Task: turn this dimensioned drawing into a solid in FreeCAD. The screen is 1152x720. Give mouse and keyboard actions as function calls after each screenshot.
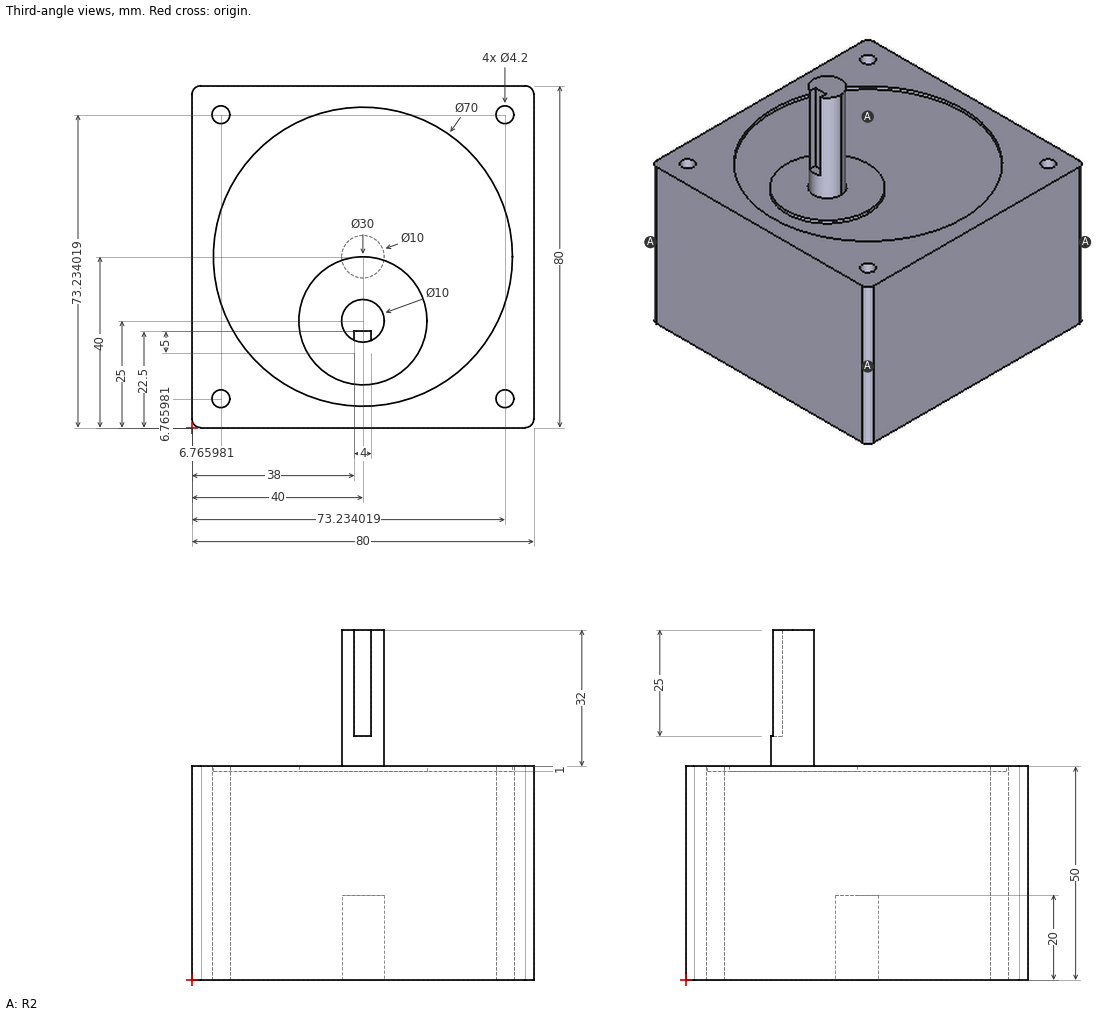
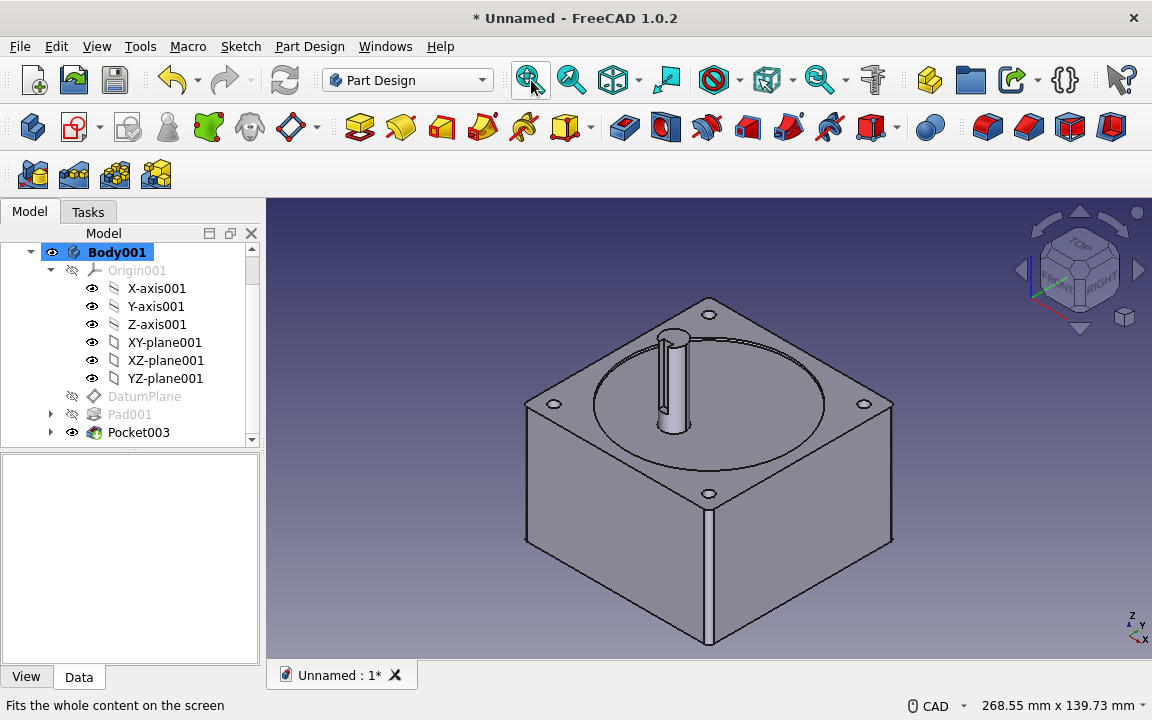
scroll(121, 338, down, 3)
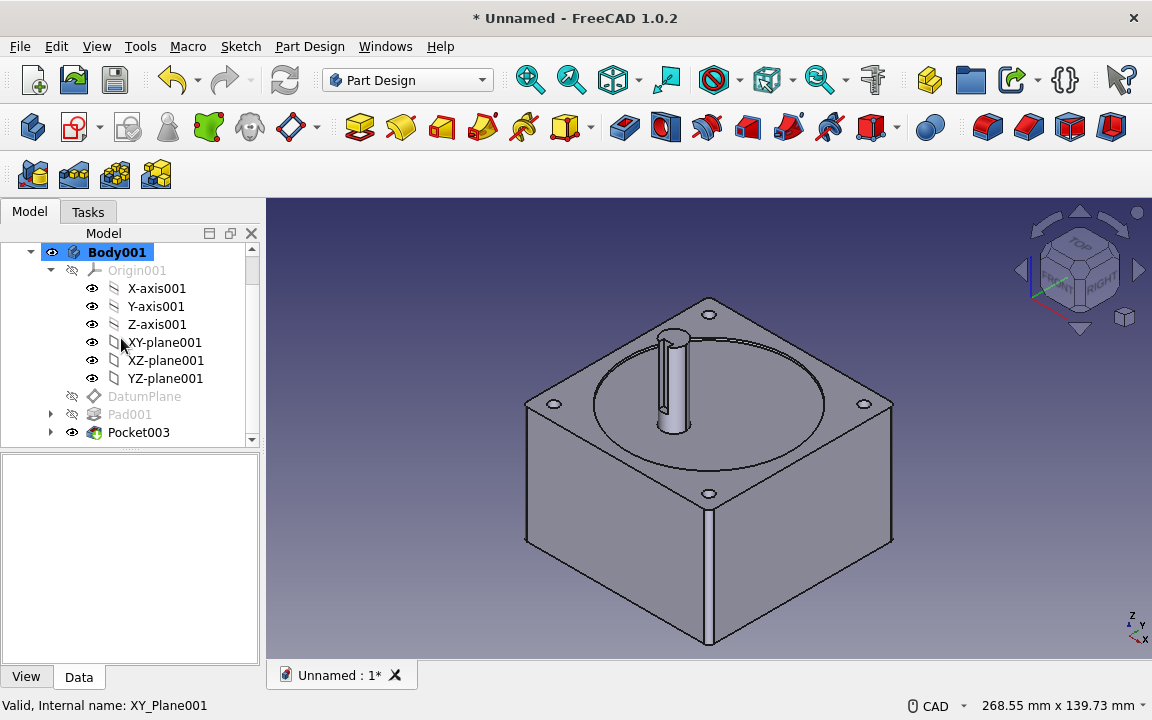
scroll(121, 338, up, 15)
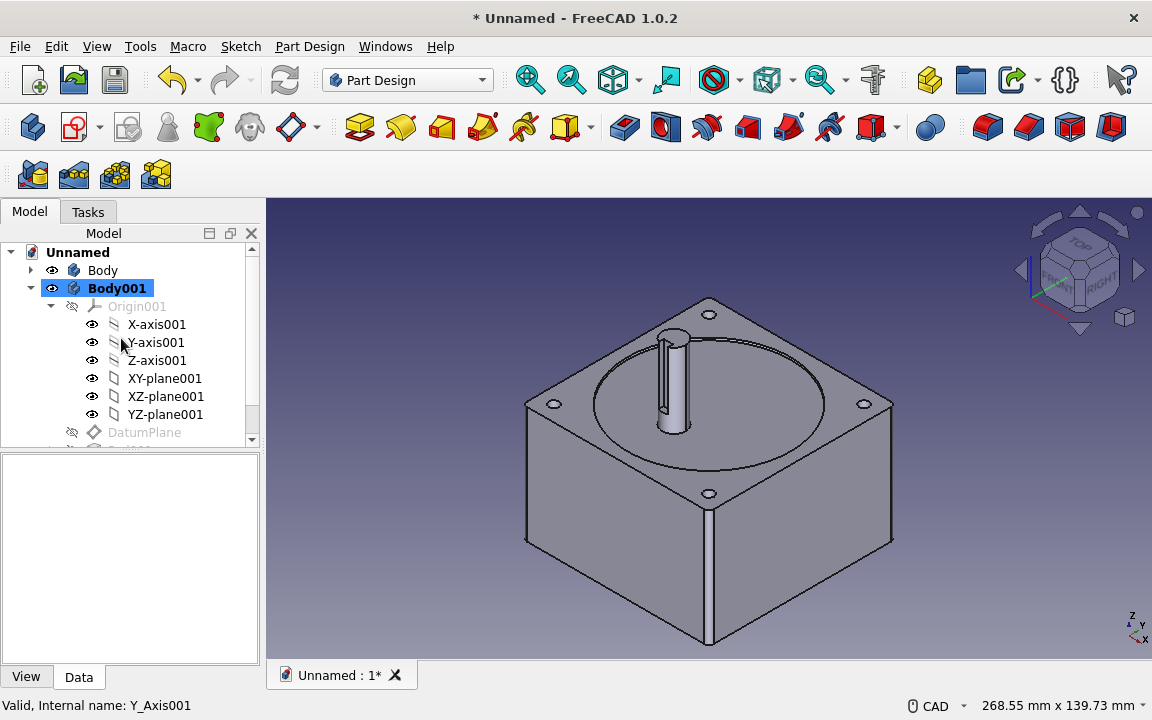
double_click(97, 270)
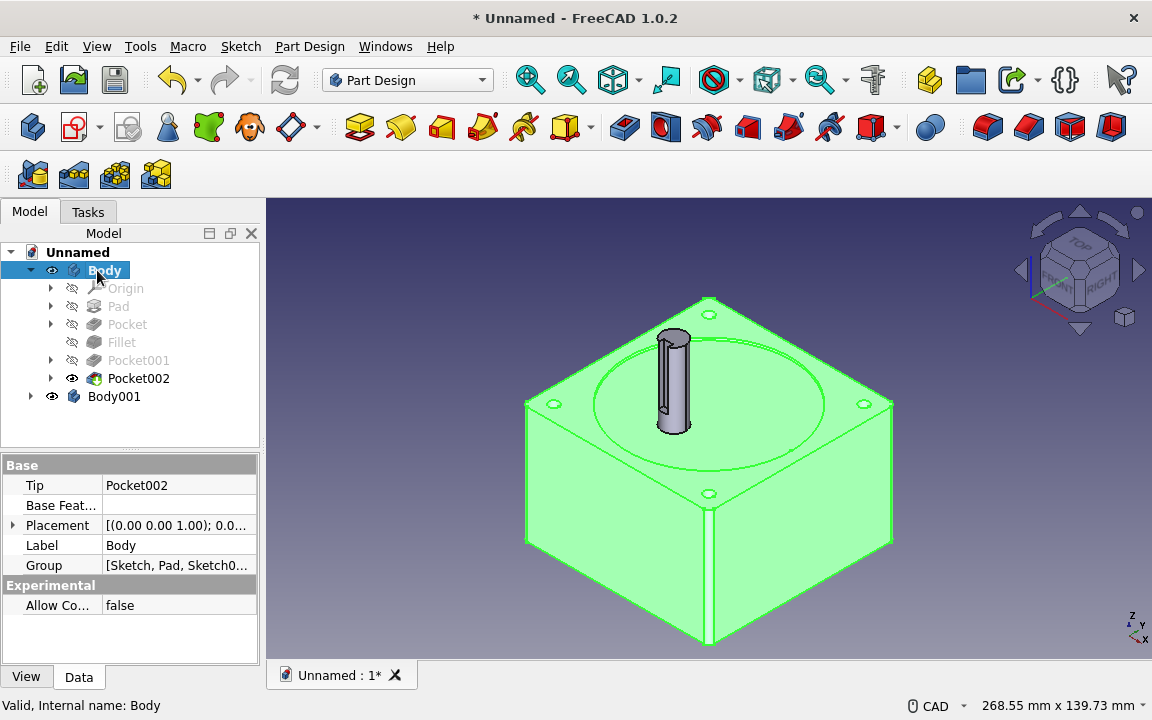
click(97, 270)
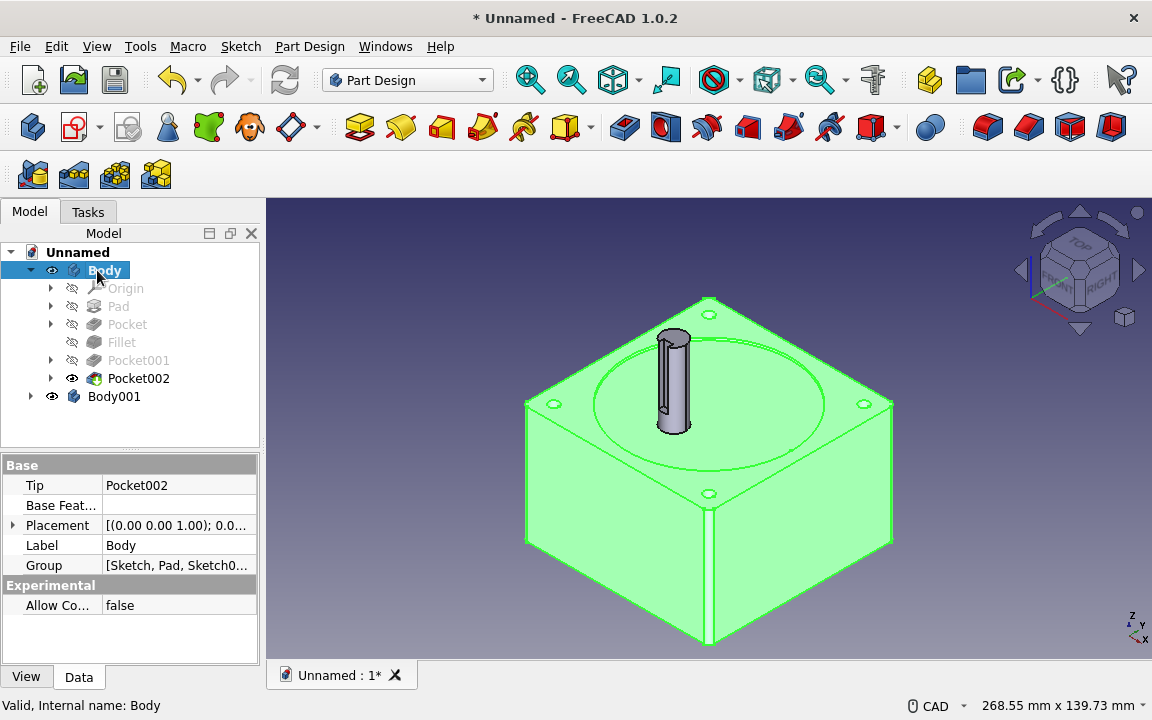
click(148, 605)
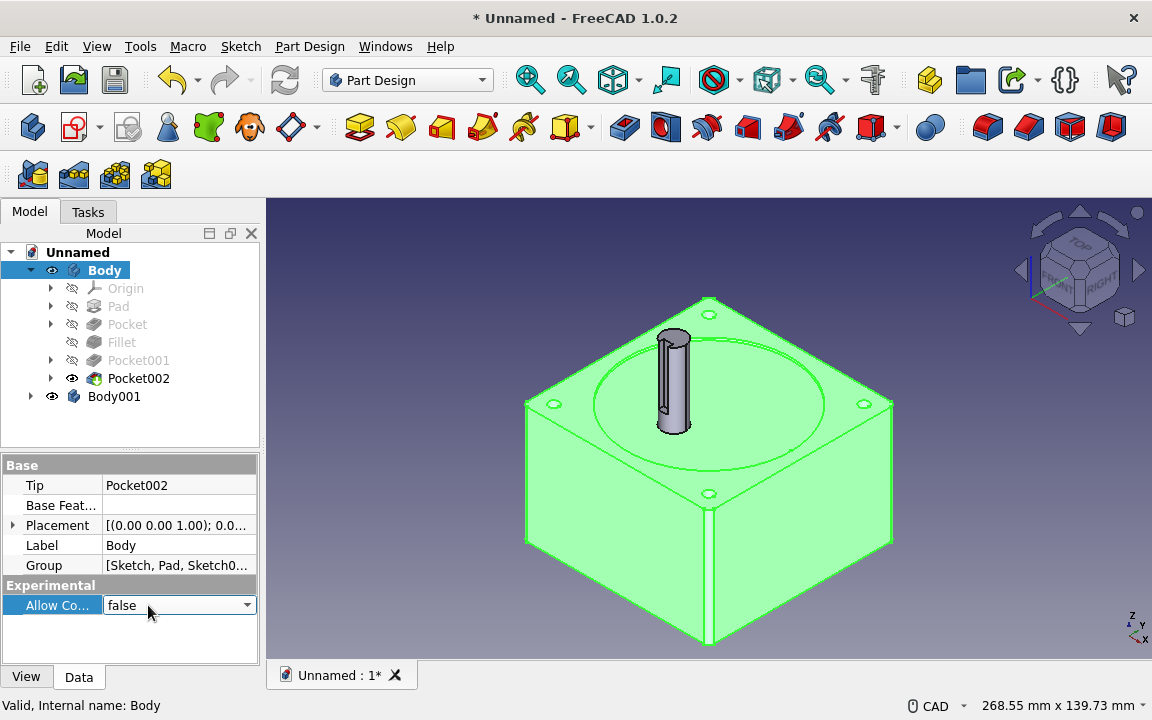
click(148, 605)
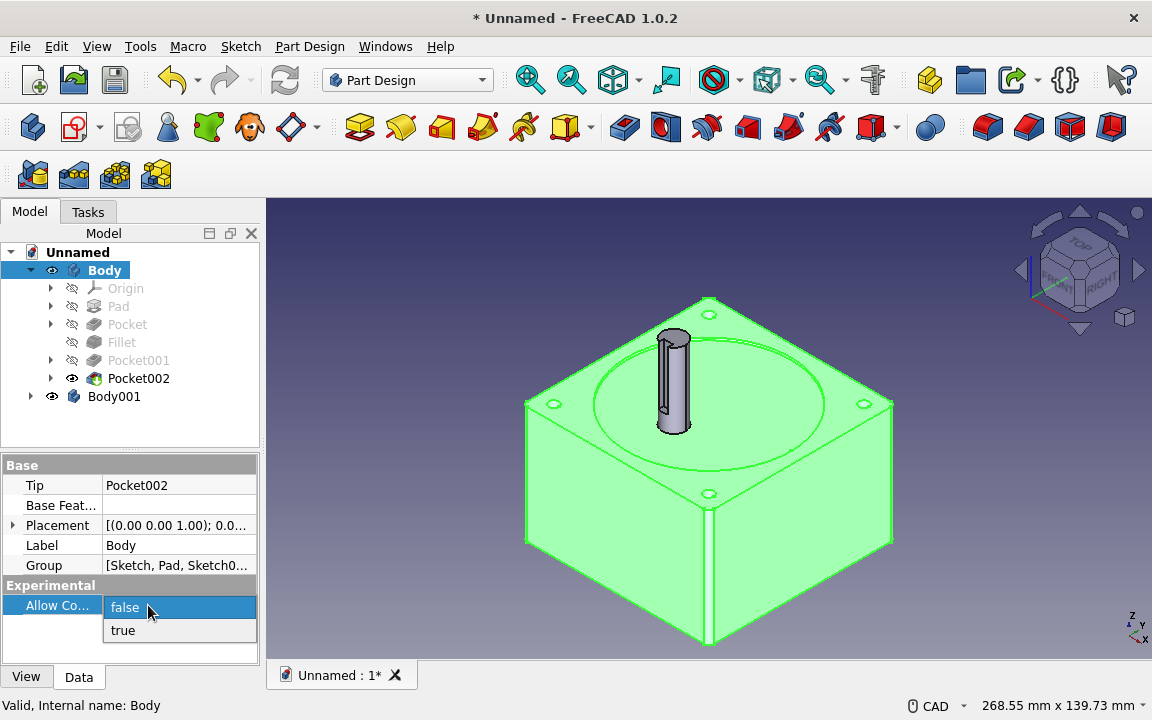
click(178, 630)
key(Return)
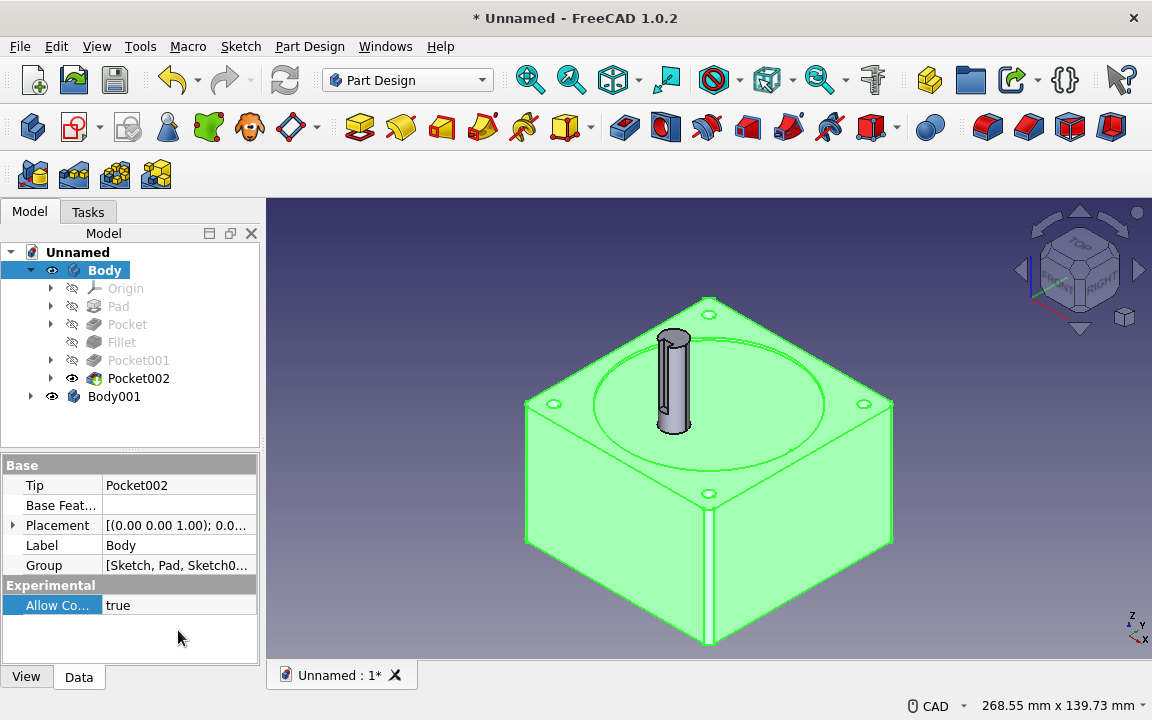
click(97, 396)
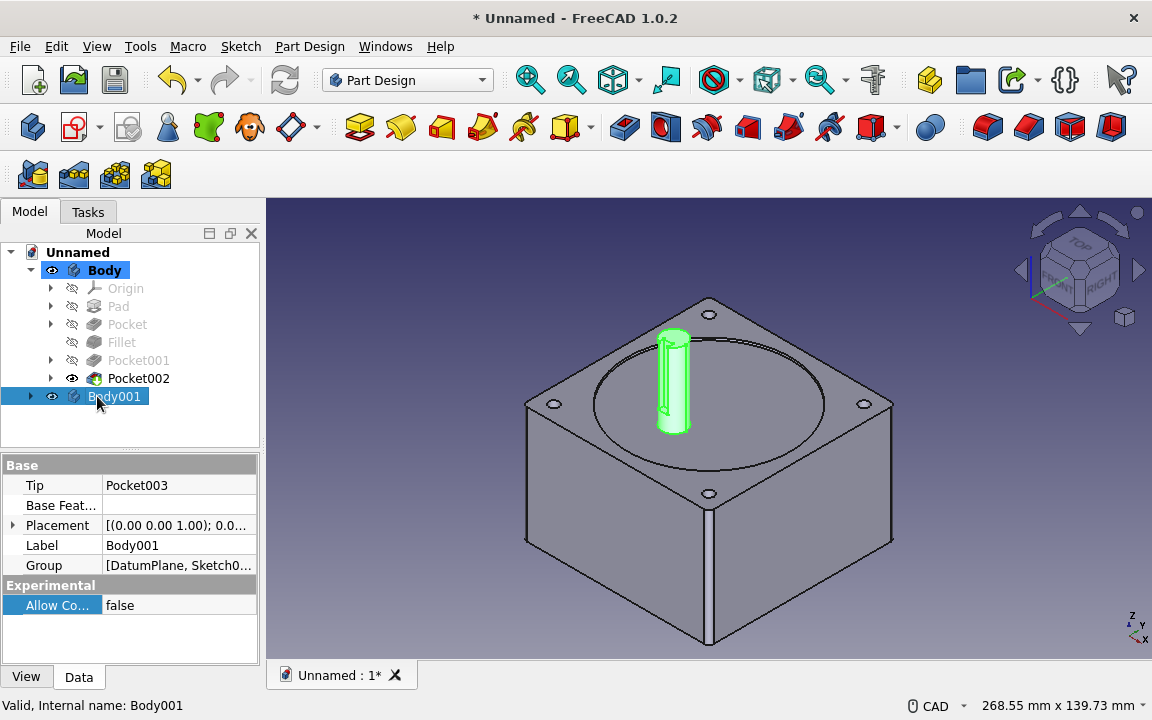
click(931, 128)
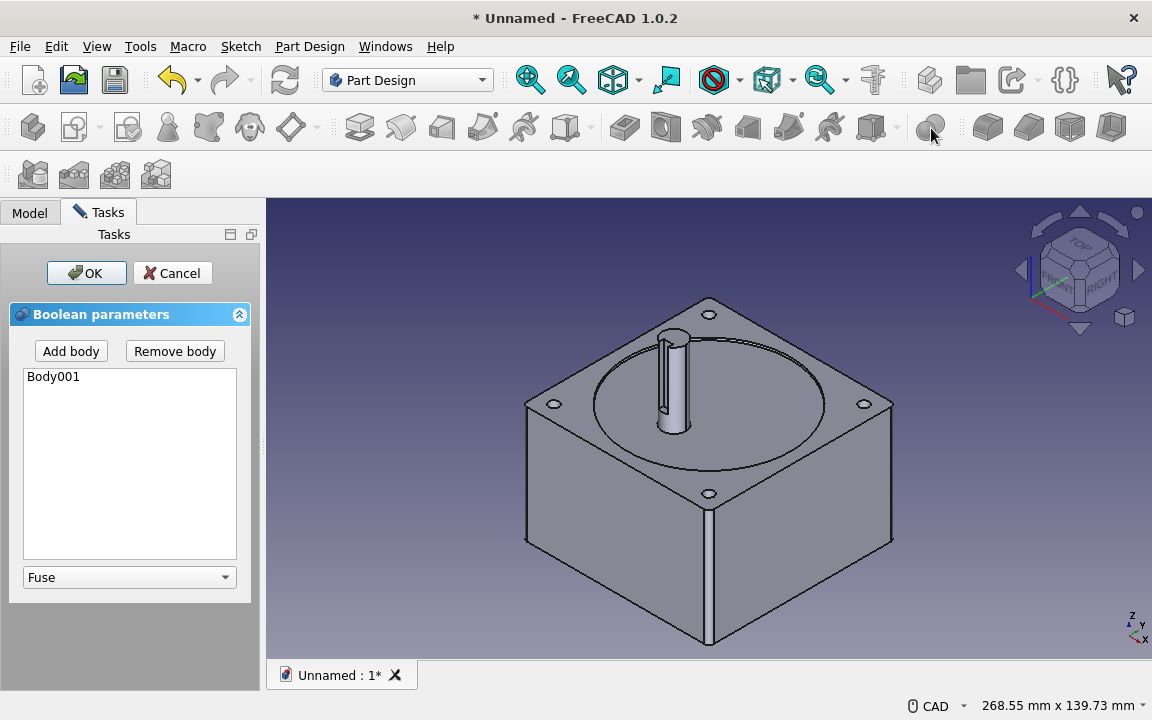
click(87, 273)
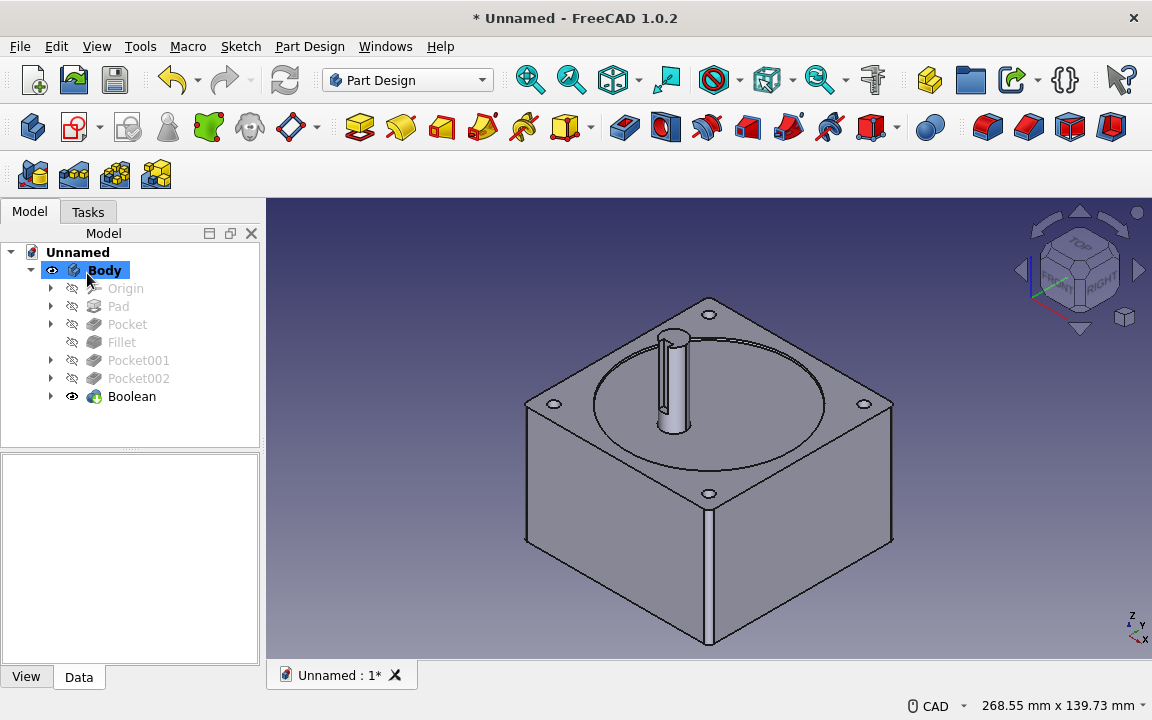
click(709, 406)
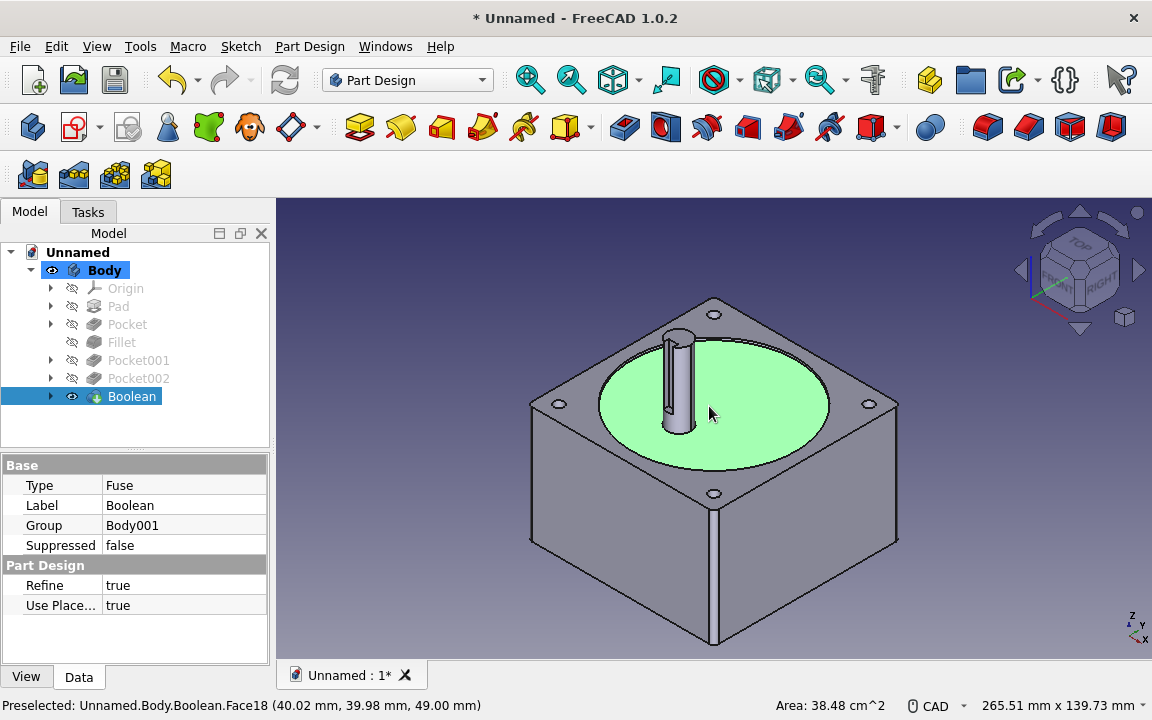
click(74, 128)